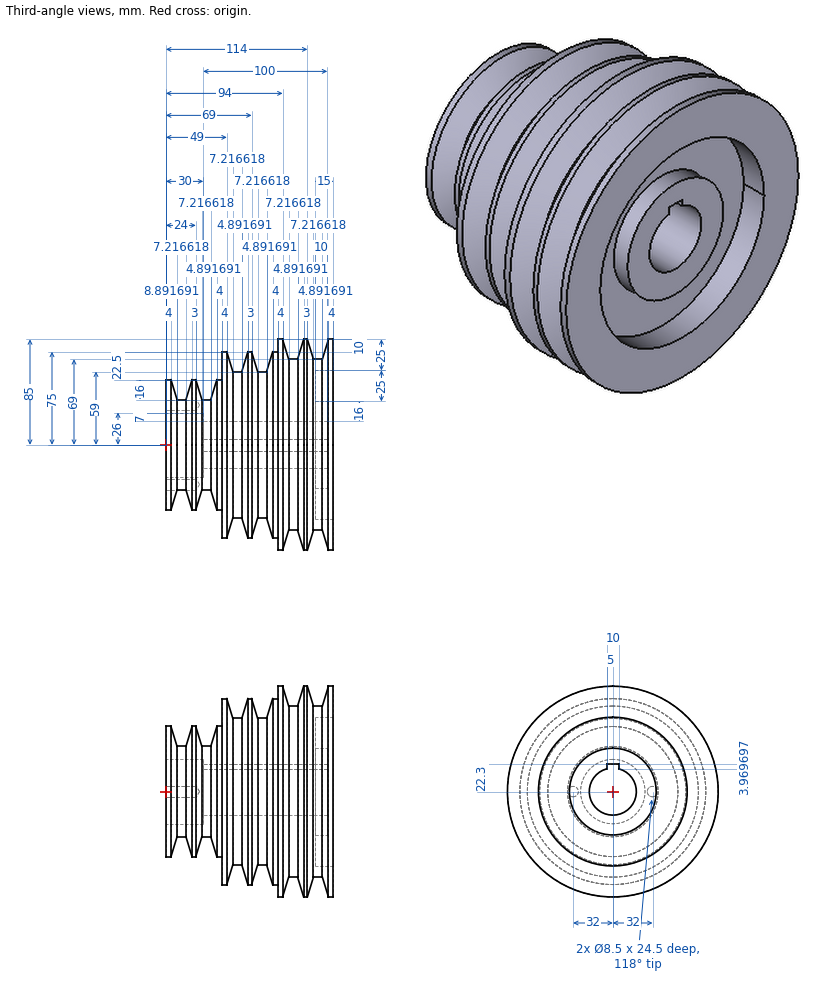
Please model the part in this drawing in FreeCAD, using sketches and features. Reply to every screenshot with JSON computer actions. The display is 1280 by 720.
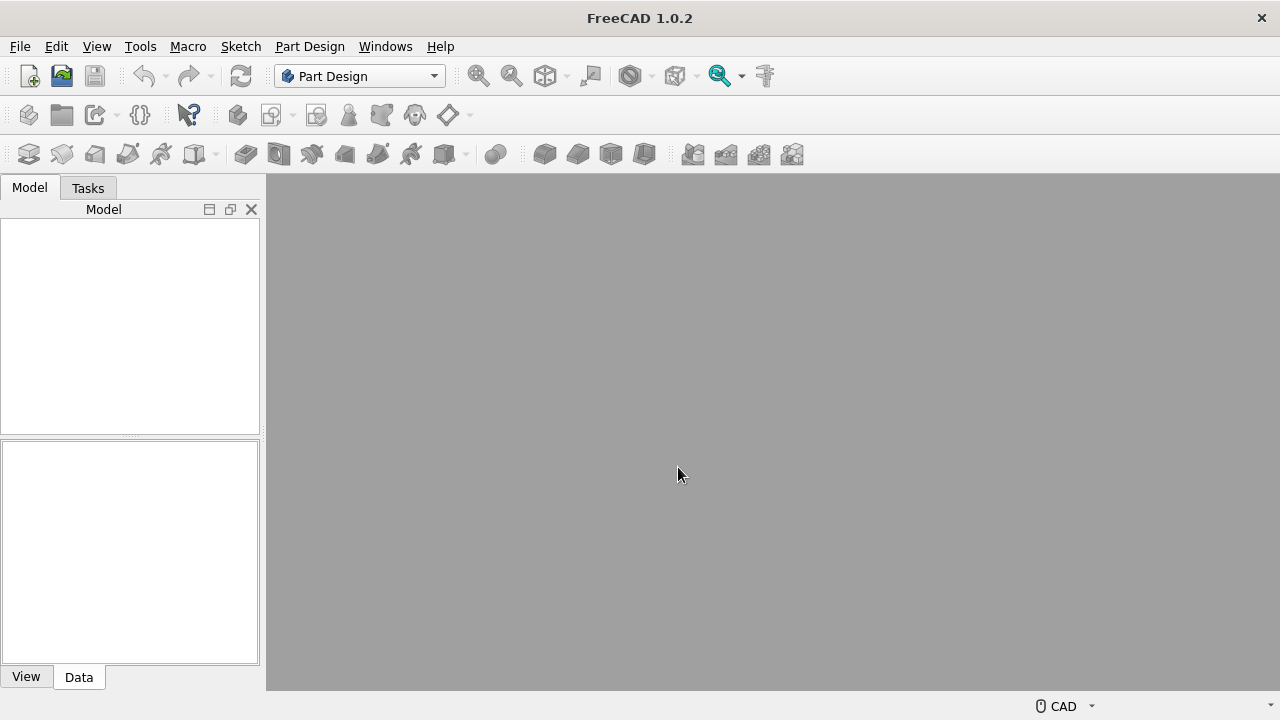
{"action": "left_click", "coordinate": [29, 76]}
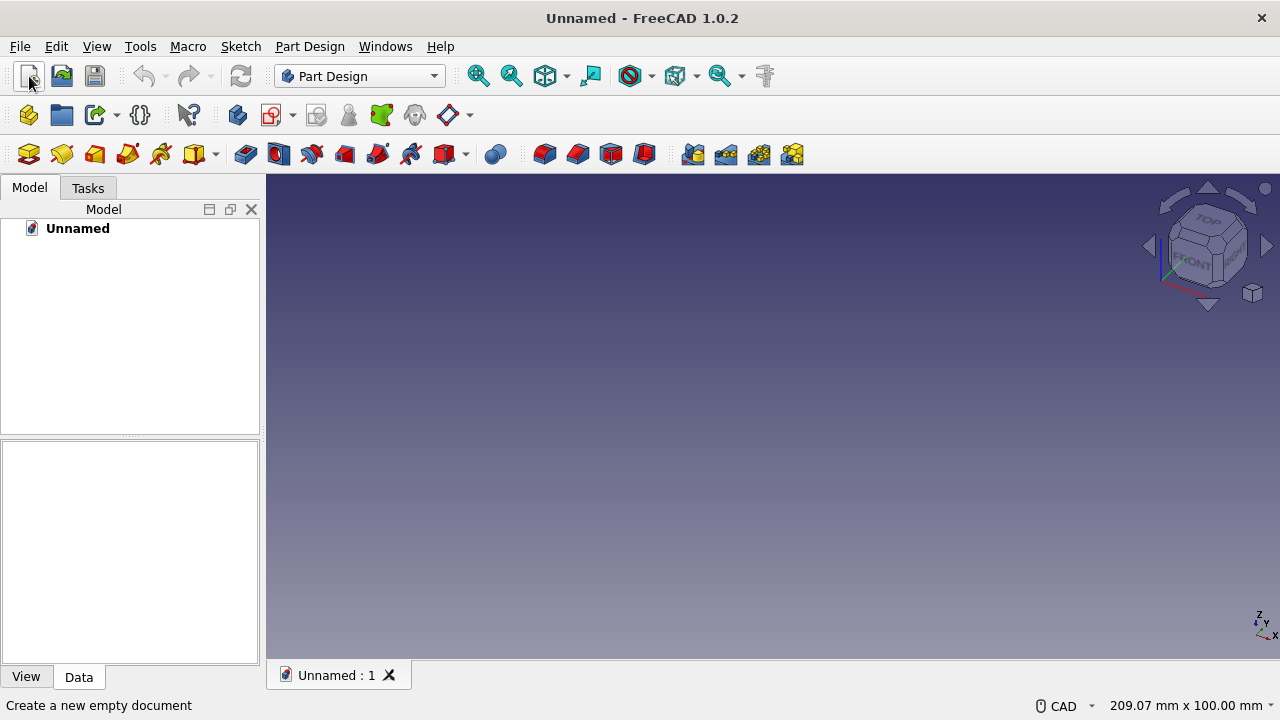
{"action": "left_click", "coordinate": [270, 116]}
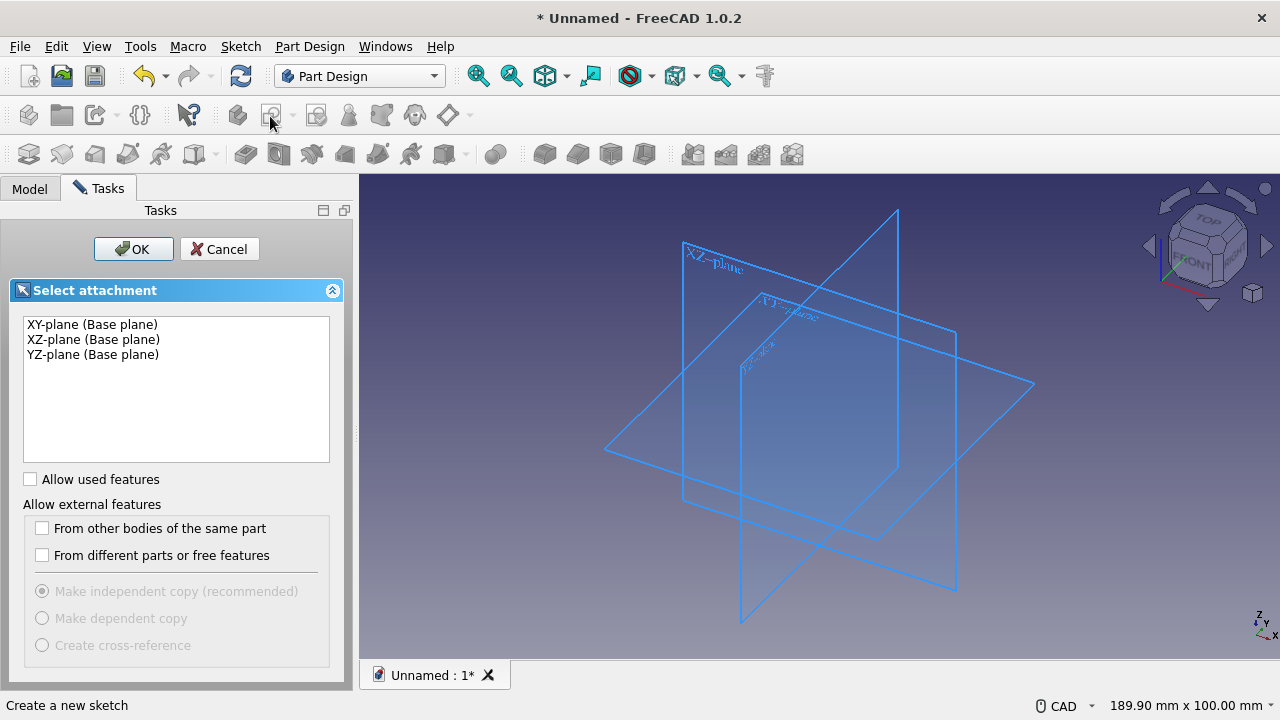
{"action": "left_click", "coordinate": [84, 324]}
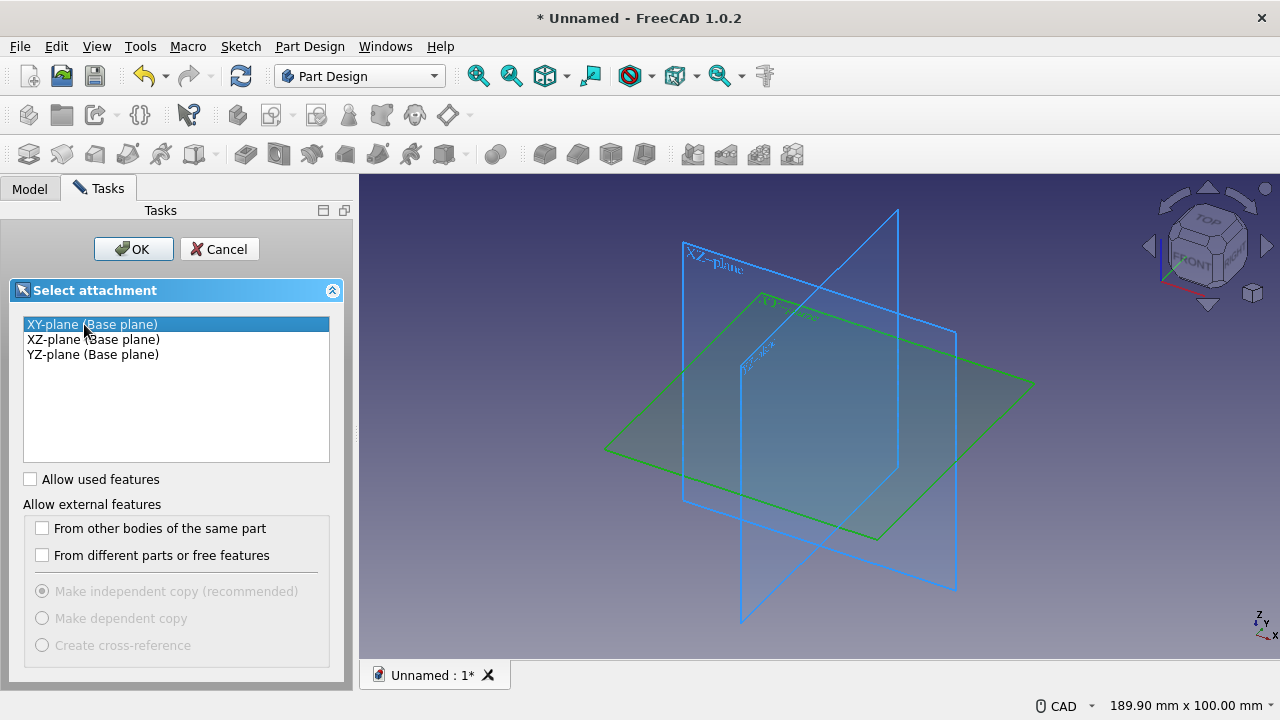
{"action": "left_click", "coordinate": [134, 249]}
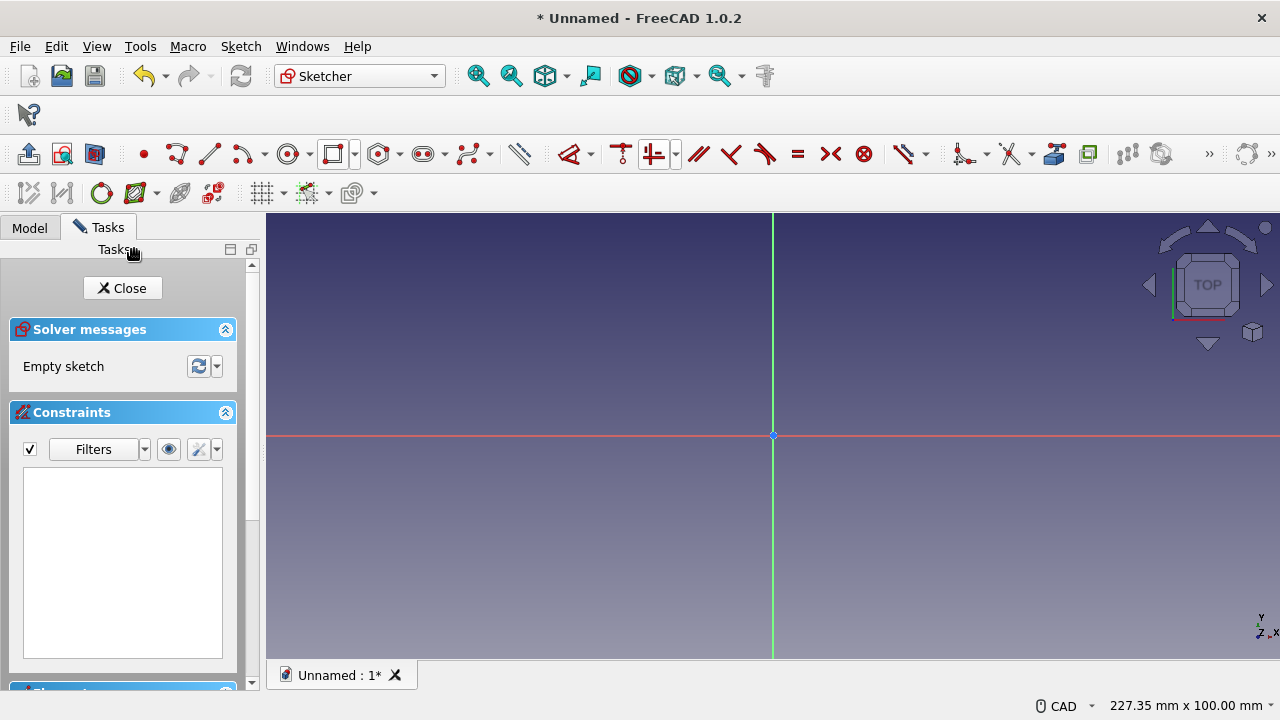
{"action": "scroll", "coordinate": [294, 631], "scroll_direction": "down", "scroll_amount": 3}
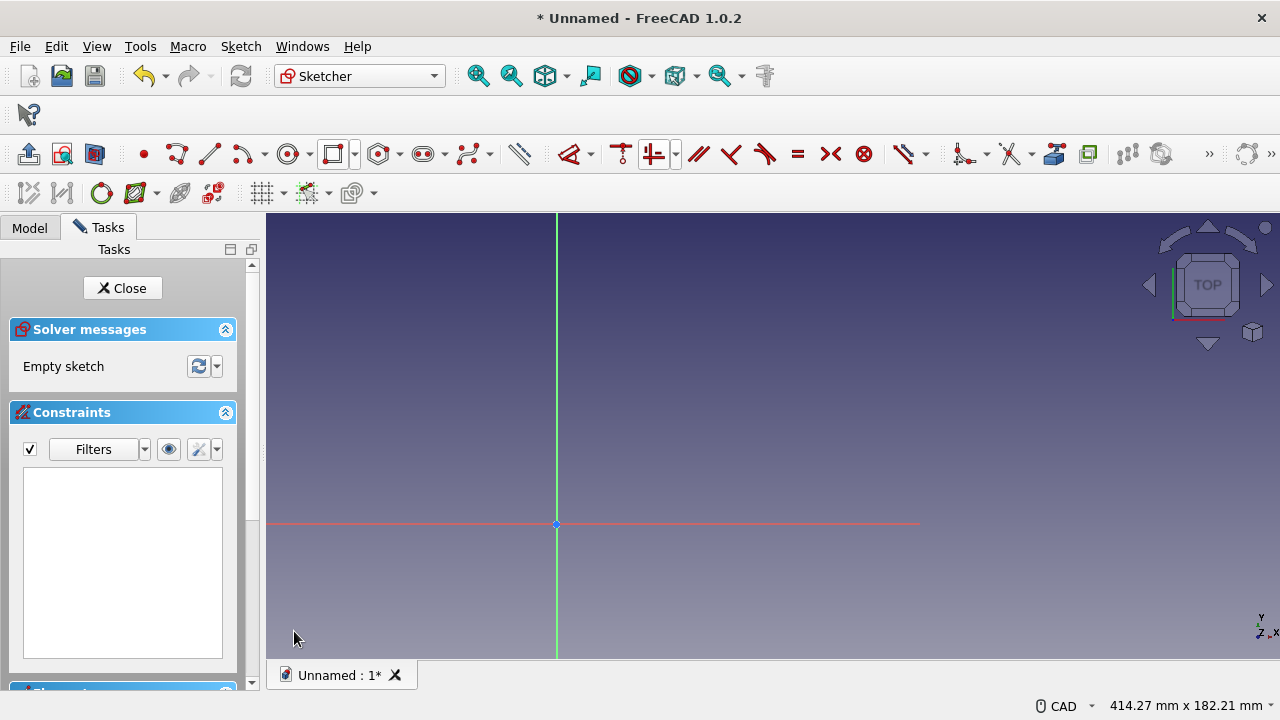
{"action": "left_click", "coordinate": [177, 154]}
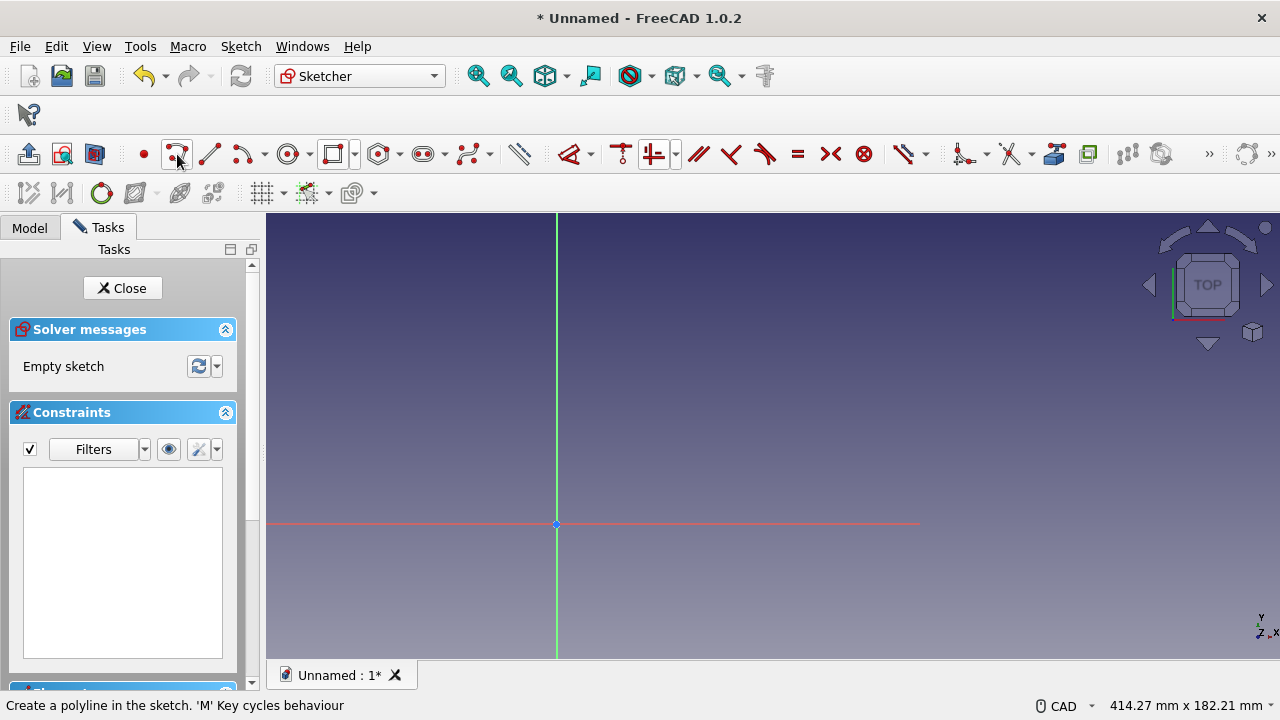
{"action": "left_click", "coordinate": [557, 461]}
{"action": "left_click", "coordinate": [630, 461]}
{"action": "left_click", "coordinate": [630, 478]}
{"action": "left_click", "coordinate": [875, 478]}
{"action": "left_click", "coordinate": [875, 439]}
{"action": "left_click", "coordinate": [851, 439]}
{"action": "left_click", "coordinate": [851, 378]}
{"action": "left_click", "coordinate": [887, 378]}
{"action": "left_click", "coordinate": [887, 316]}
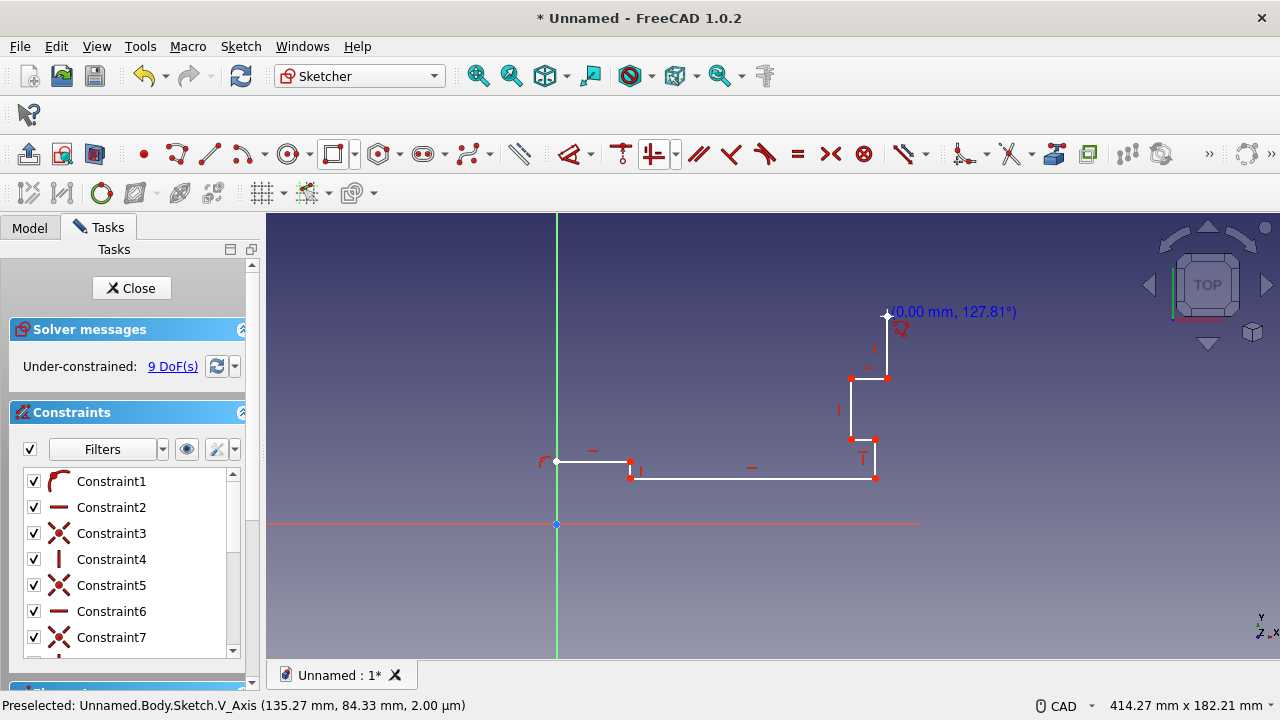
{"action": "scroll", "coordinate": [878, 316], "scroll_direction": "up", "scroll_amount": 3}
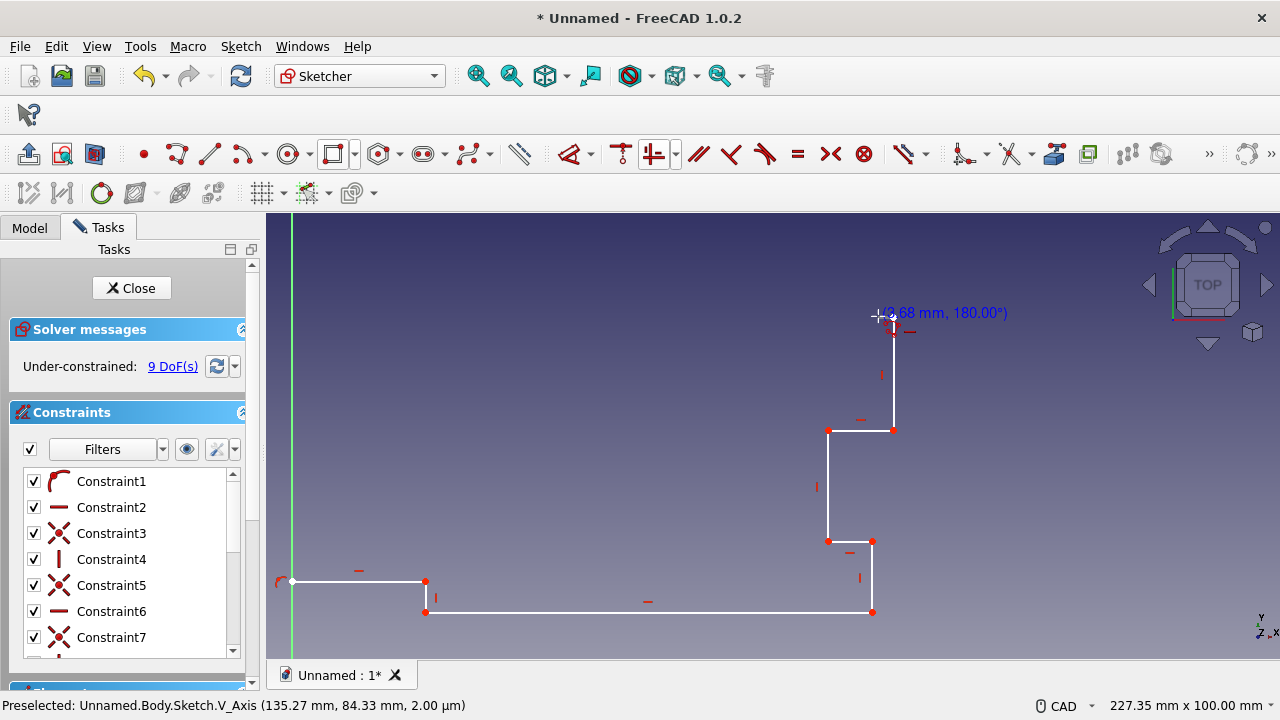
{"action": "left_click", "coordinate": [877, 316]}
{"action": "left_click", "coordinate": [855, 388]}
{"action": "left_click", "coordinate": [823, 388]}
{"action": "left_click", "coordinate": [801, 316]}
{"action": "left_click", "coordinate": [787, 316]}
{"action": "left_click", "coordinate": [766, 388]}
{"action": "left_click", "coordinate": [733, 388]}
{"action": "left_click", "coordinate": [712, 316]}
{"action": "left_click", "coordinate": [694, 316]}
{"action": "left_click", "coordinate": [694, 361]}
{"action": "left_click", "coordinate": [676, 361]}
{"action": "left_click", "coordinate": [654, 432]}
{"action": "left_click", "coordinate": [622, 432]}
{"action": "left_click", "coordinate": [600, 361]}
{"action": "left_click", "coordinate": [587, 361]}
{"action": "left_click", "coordinate": [565, 432]}
{"action": "left_click", "coordinate": [533, 432]}
{"action": "left_click", "coordinate": [511, 361]}
{"action": "left_click", "coordinate": [493, 361]}
{"action": "left_click", "coordinate": [493, 461]}
{"action": "left_click", "coordinate": [475, 461]}
{"action": "left_click", "coordinate": [453, 533]}
{"action": "left_click", "coordinate": [421, 533]}
{"action": "left_click", "coordinate": [399, 461]}
{"action": "left_click", "coordinate": [386, 461]}
{"action": "left_click", "coordinate": [364, 533]}
{"action": "left_click", "coordinate": [332, 533]}
{"action": "left_click", "coordinate": [310, 461]}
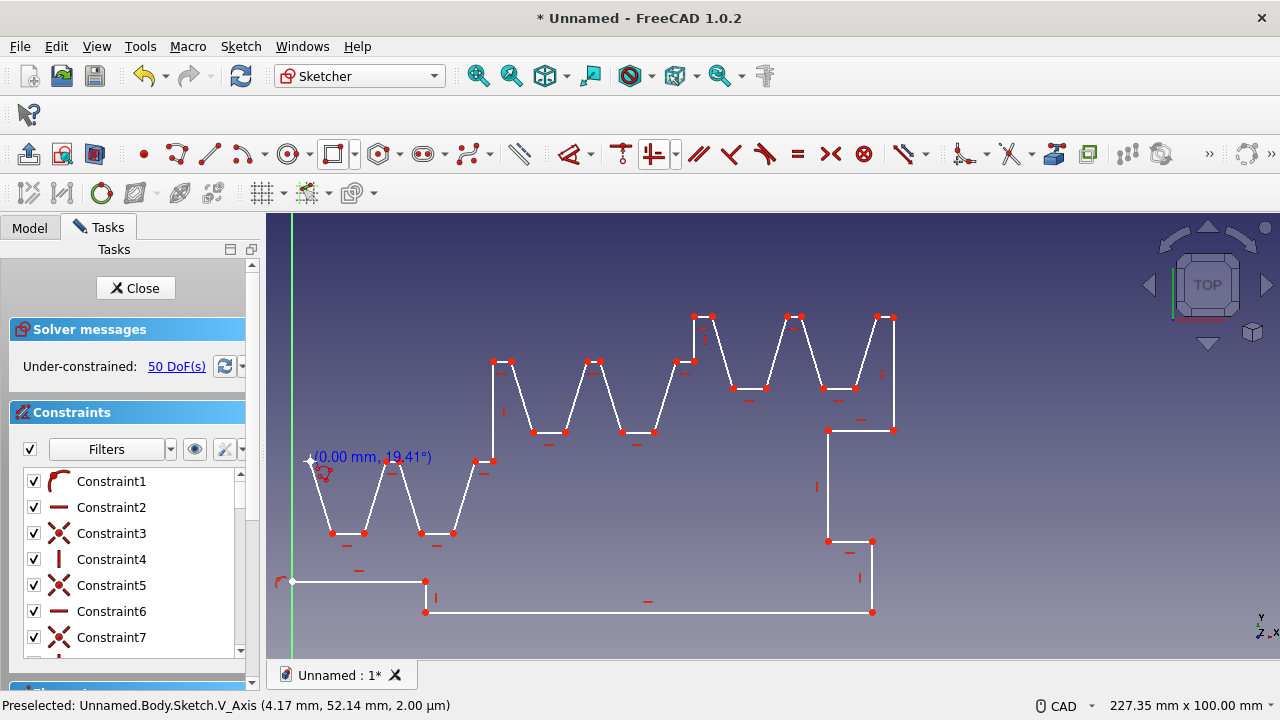
{"action": "scroll", "coordinate": [930, 294], "scroll_direction": "down", "scroll_amount": 2}